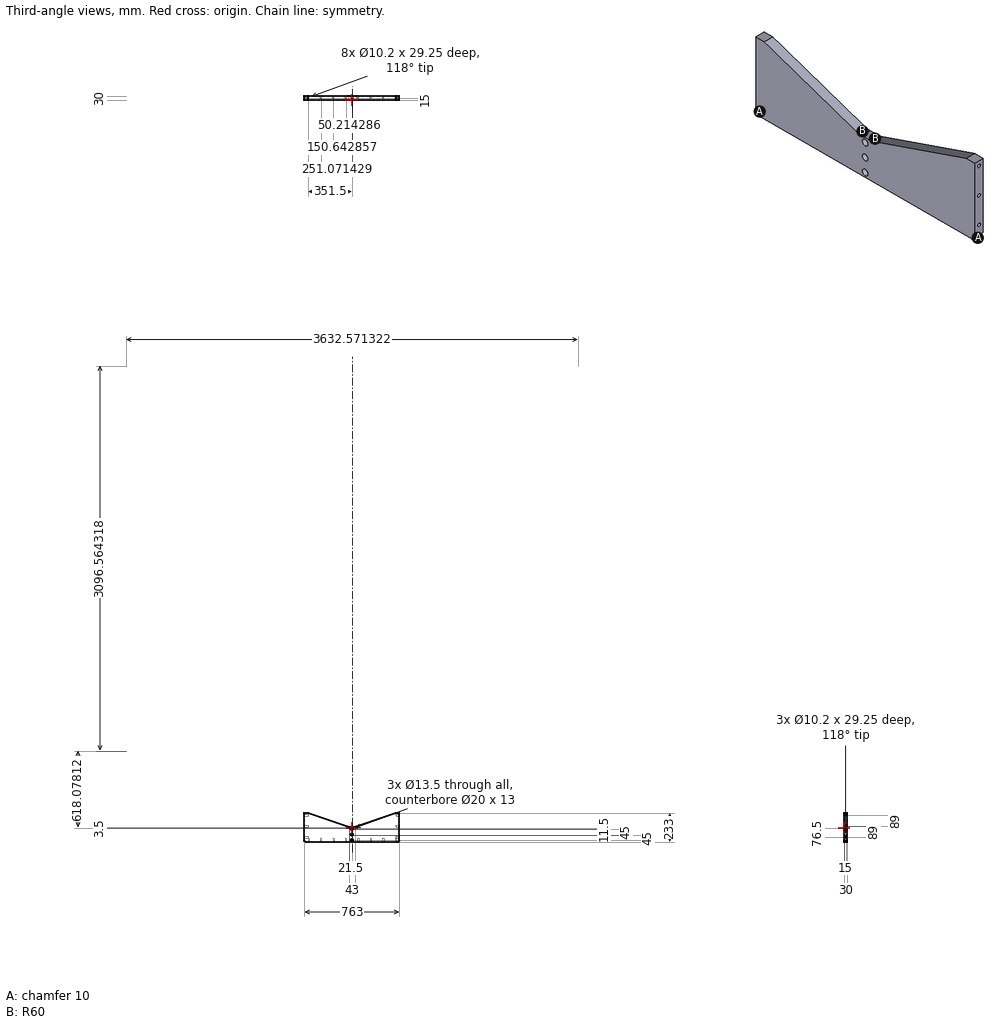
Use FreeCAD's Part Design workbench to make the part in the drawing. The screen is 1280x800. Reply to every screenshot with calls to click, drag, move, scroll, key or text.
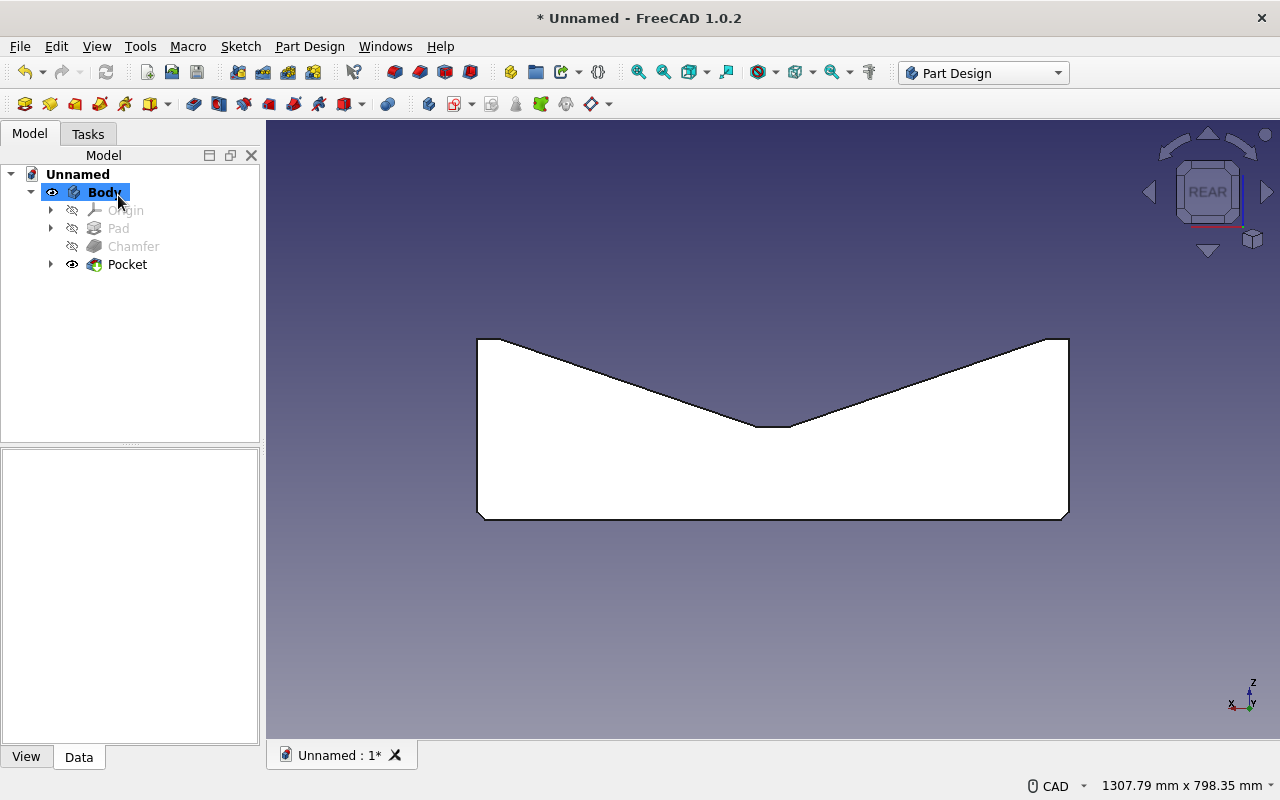
key(6)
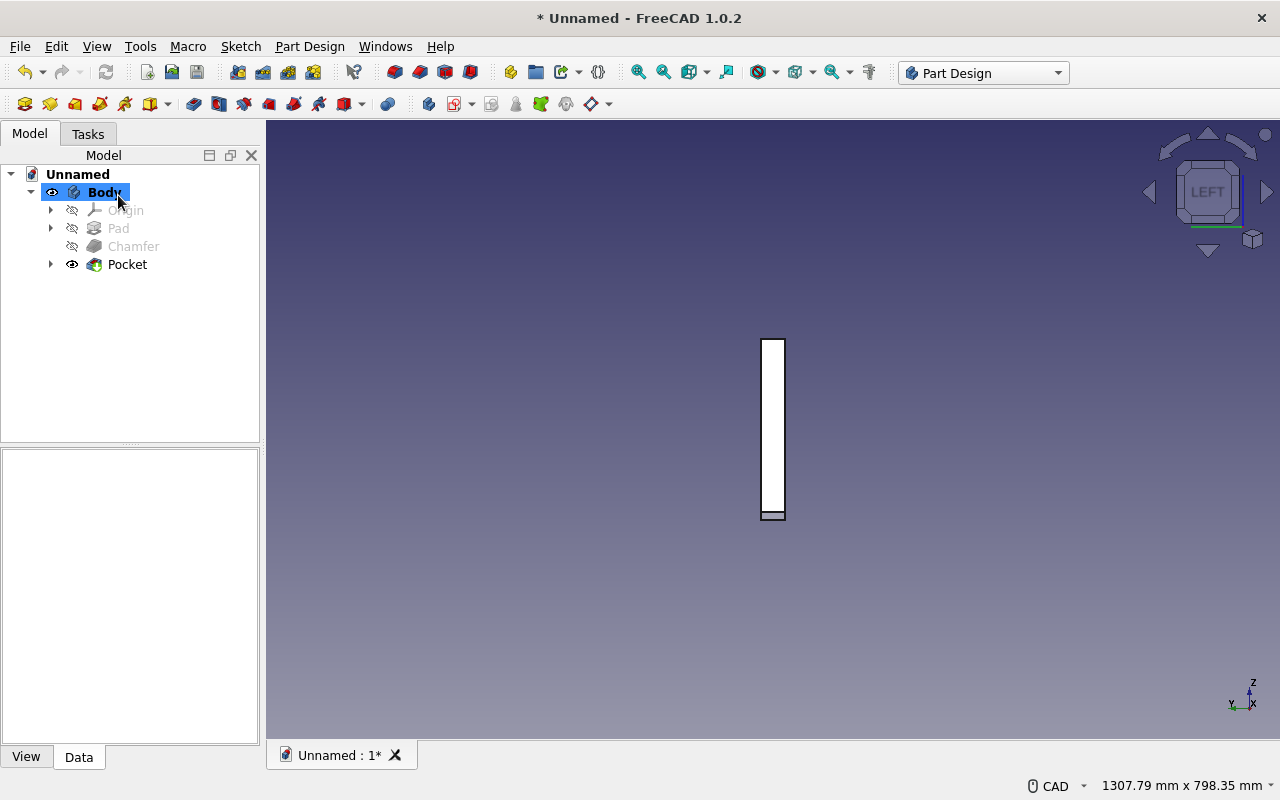
key(v)
key(f)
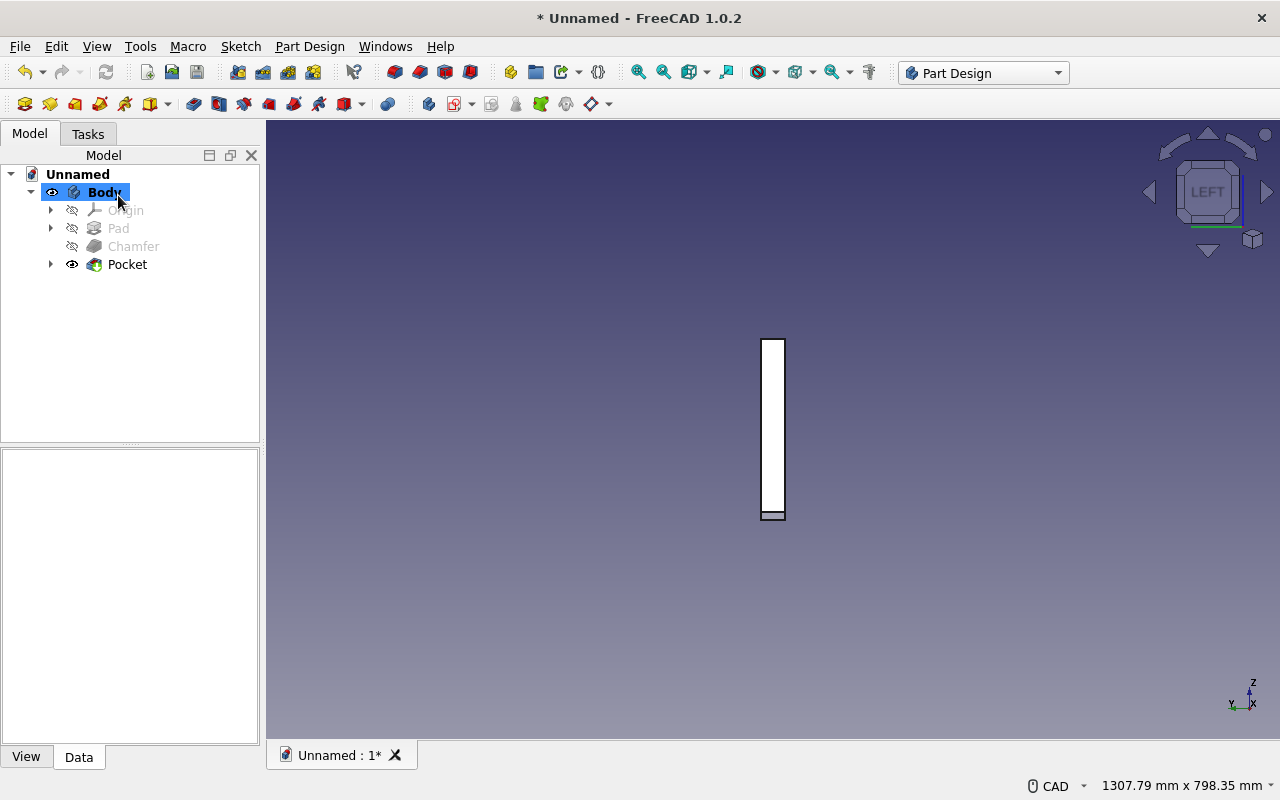
key(v)
key(3)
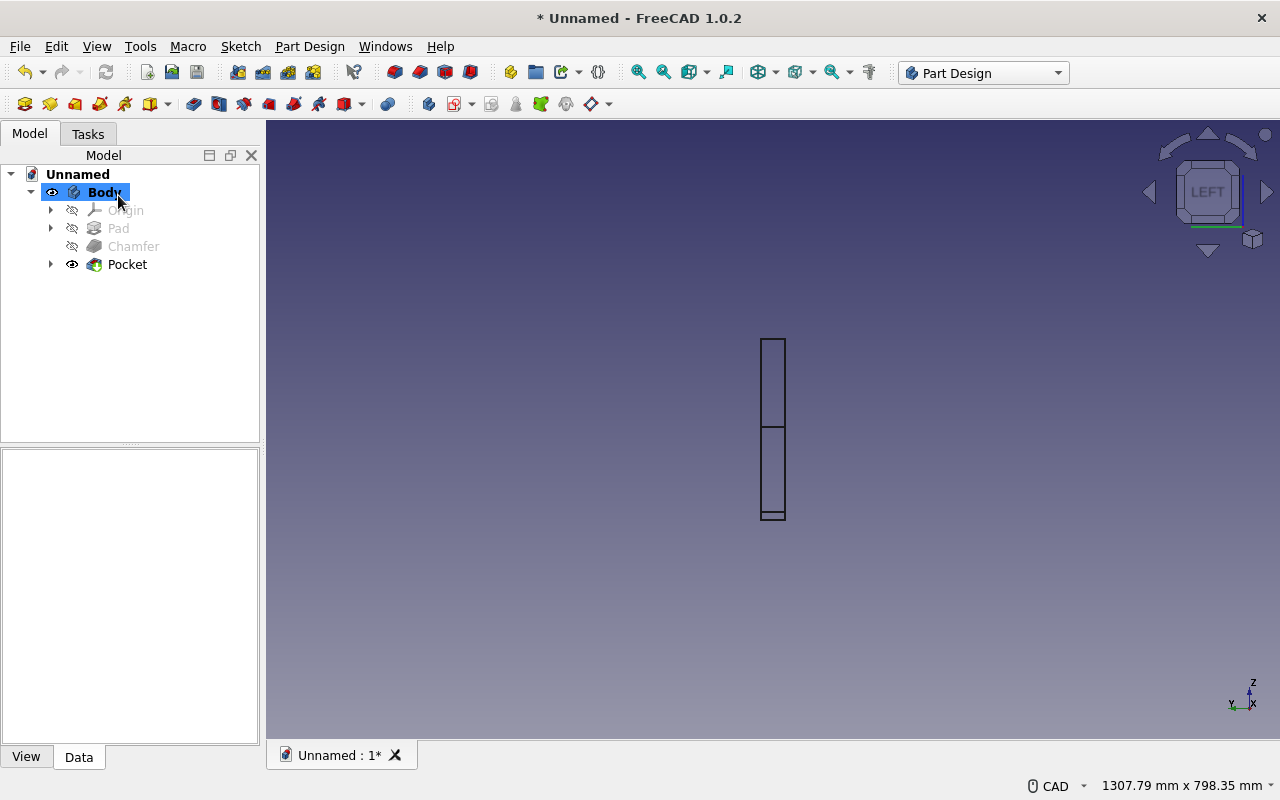
key(0)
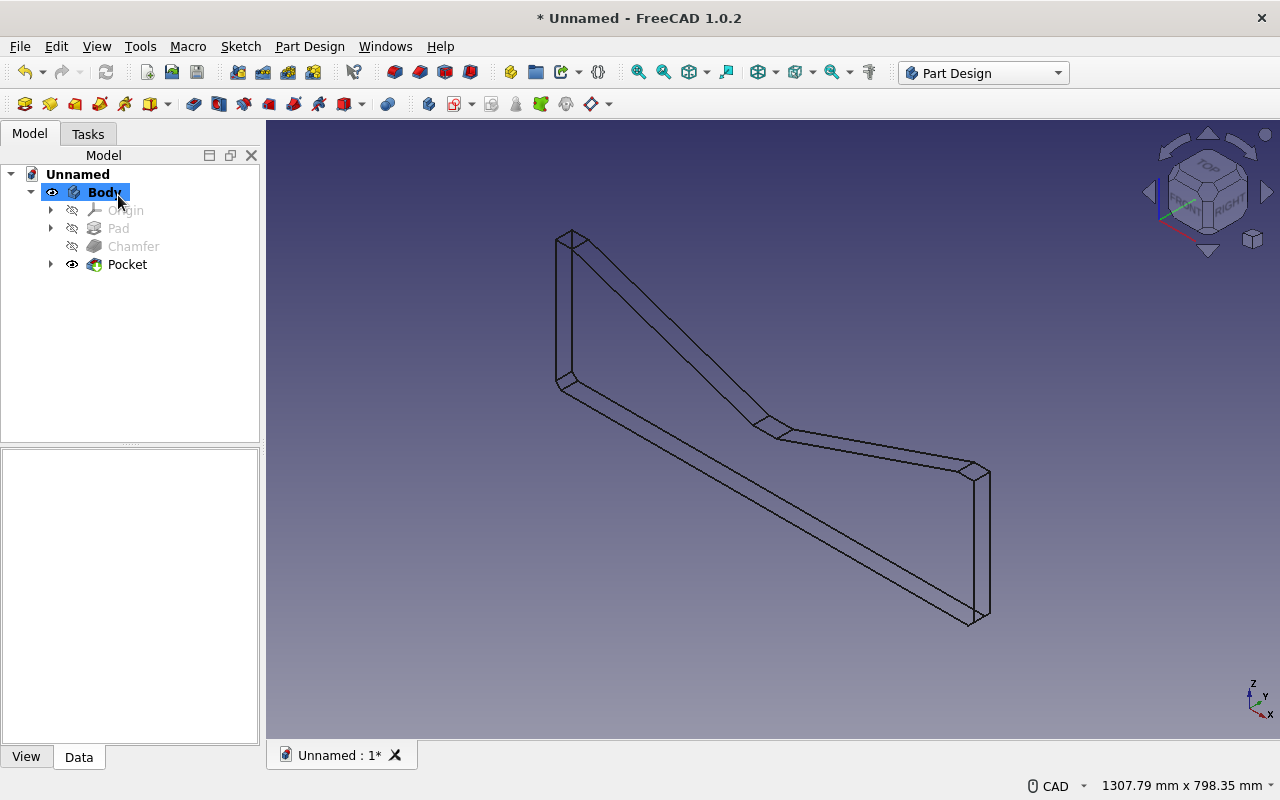
click(785, 433)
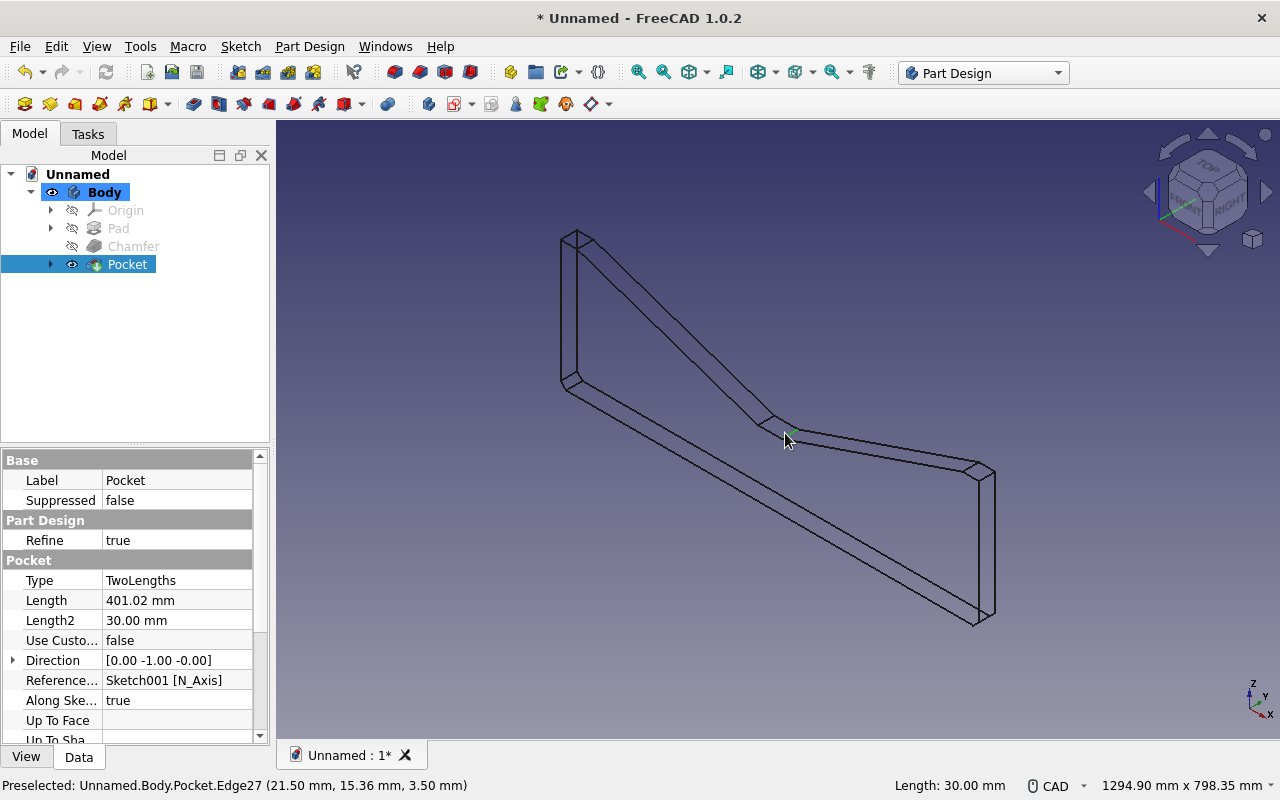
click(766, 419, ctrl)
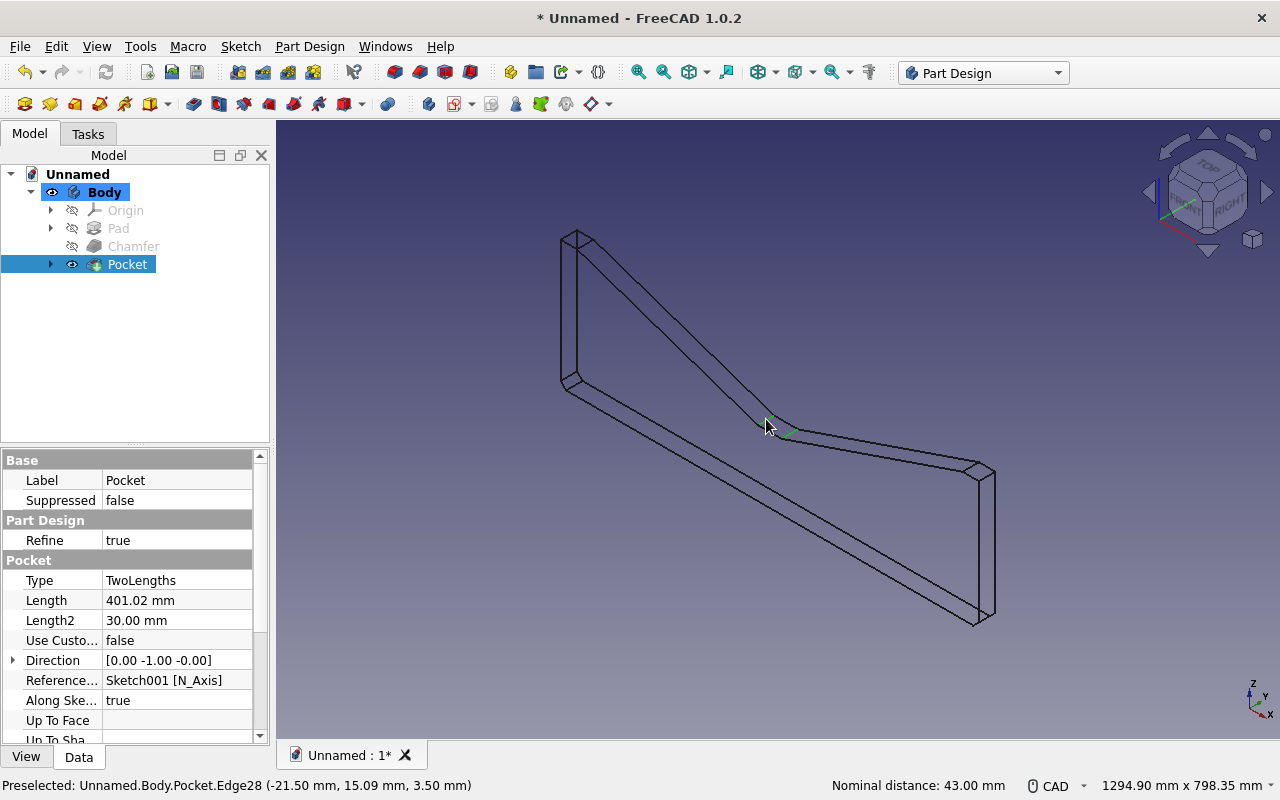
key(v)
key(1)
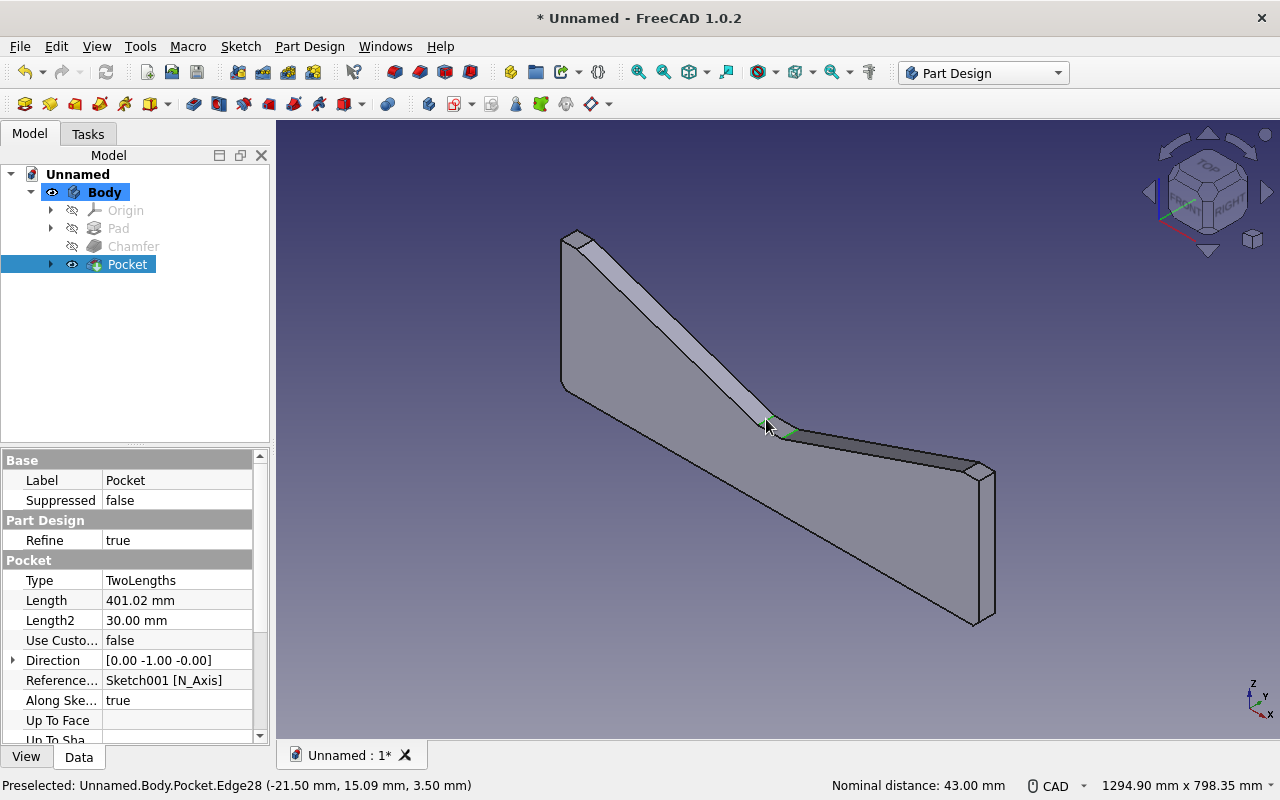
click(395, 72)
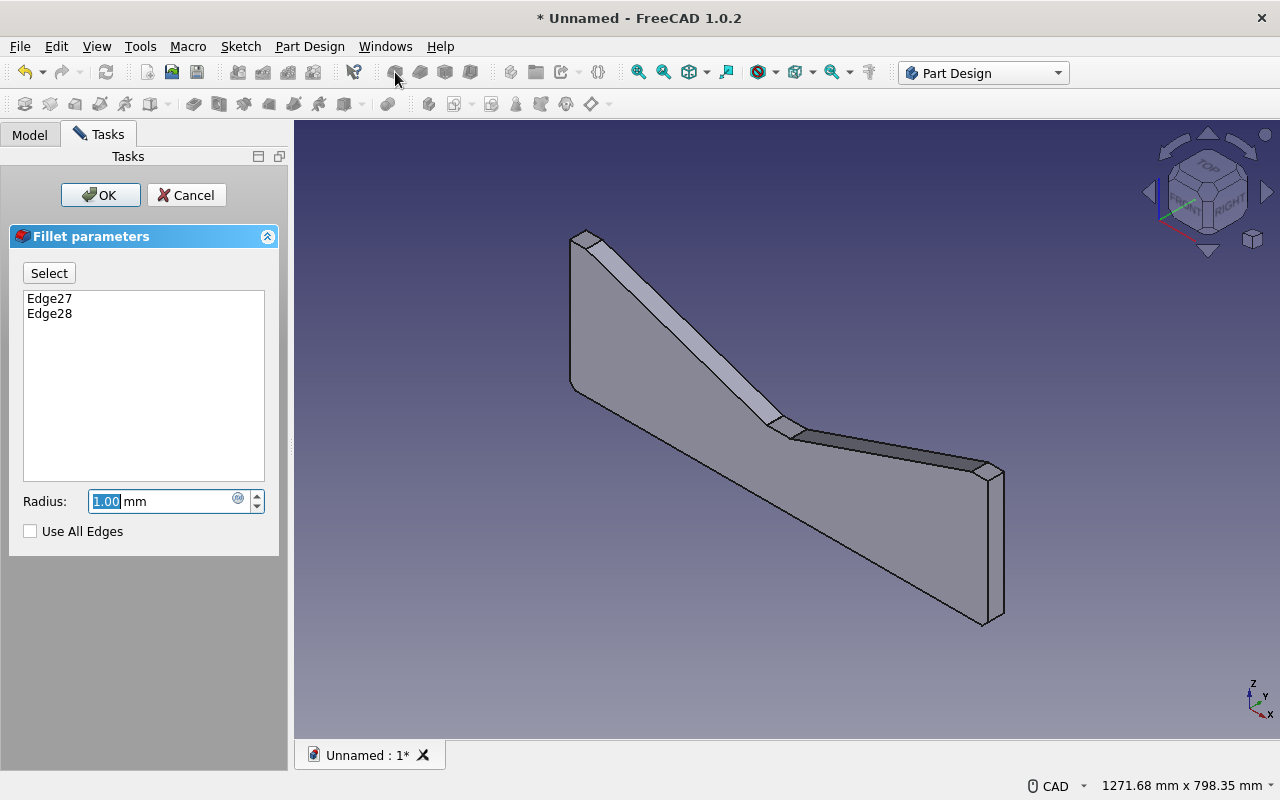
text(60)
key(Tab)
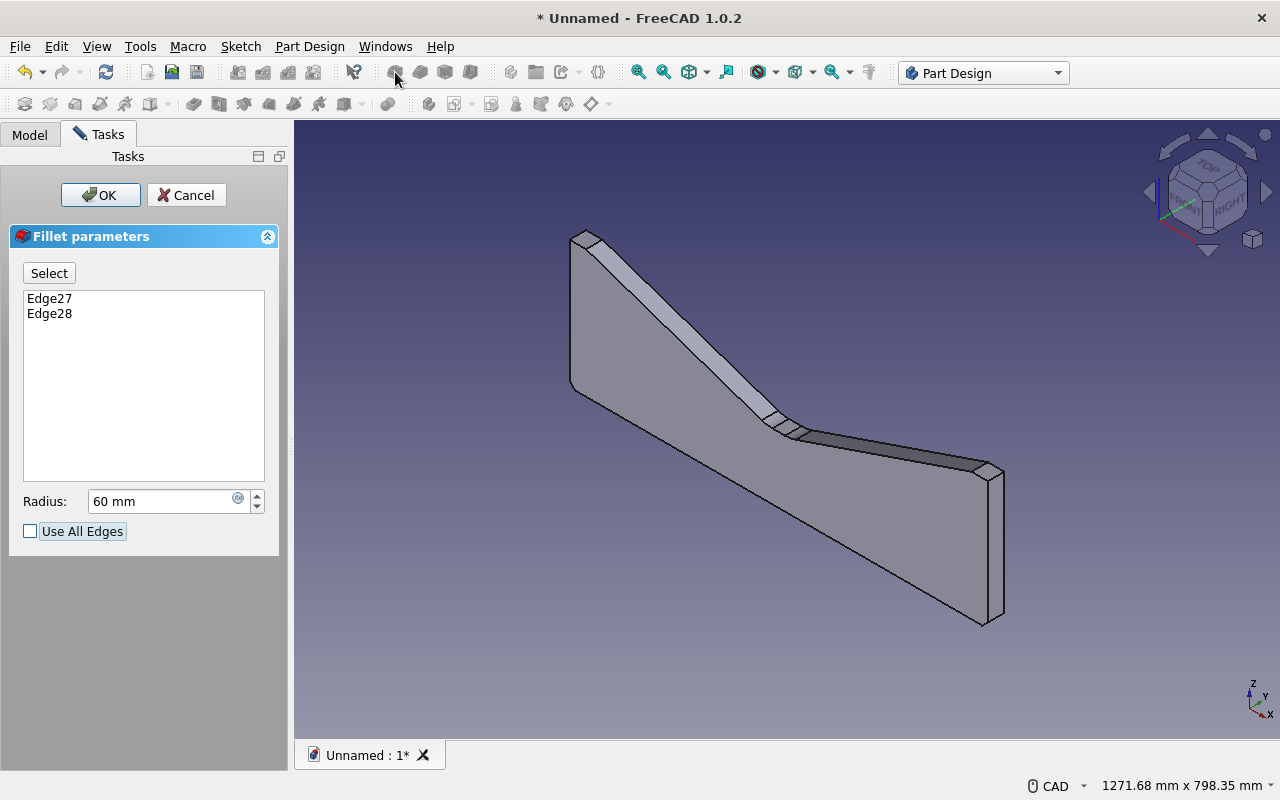
click(101, 195)